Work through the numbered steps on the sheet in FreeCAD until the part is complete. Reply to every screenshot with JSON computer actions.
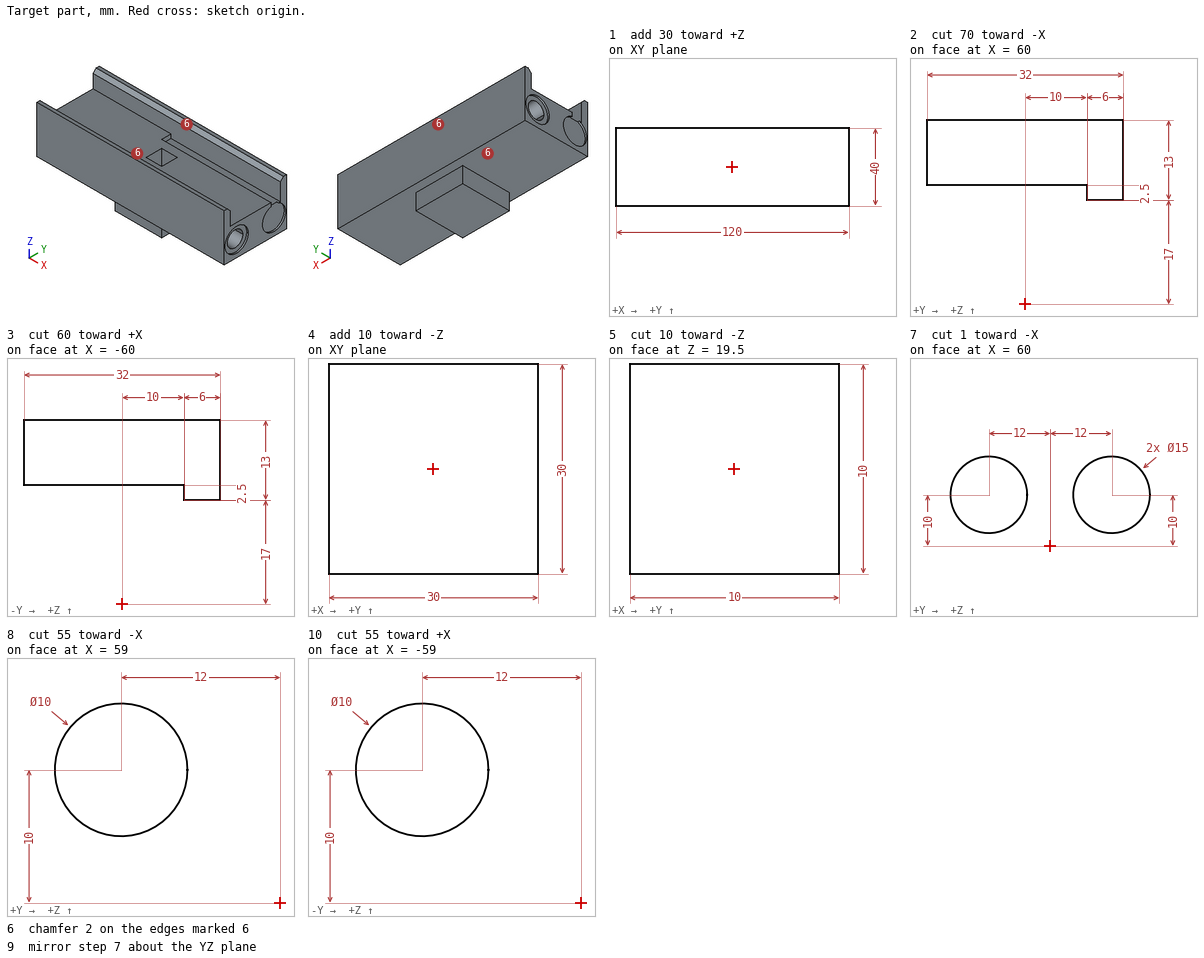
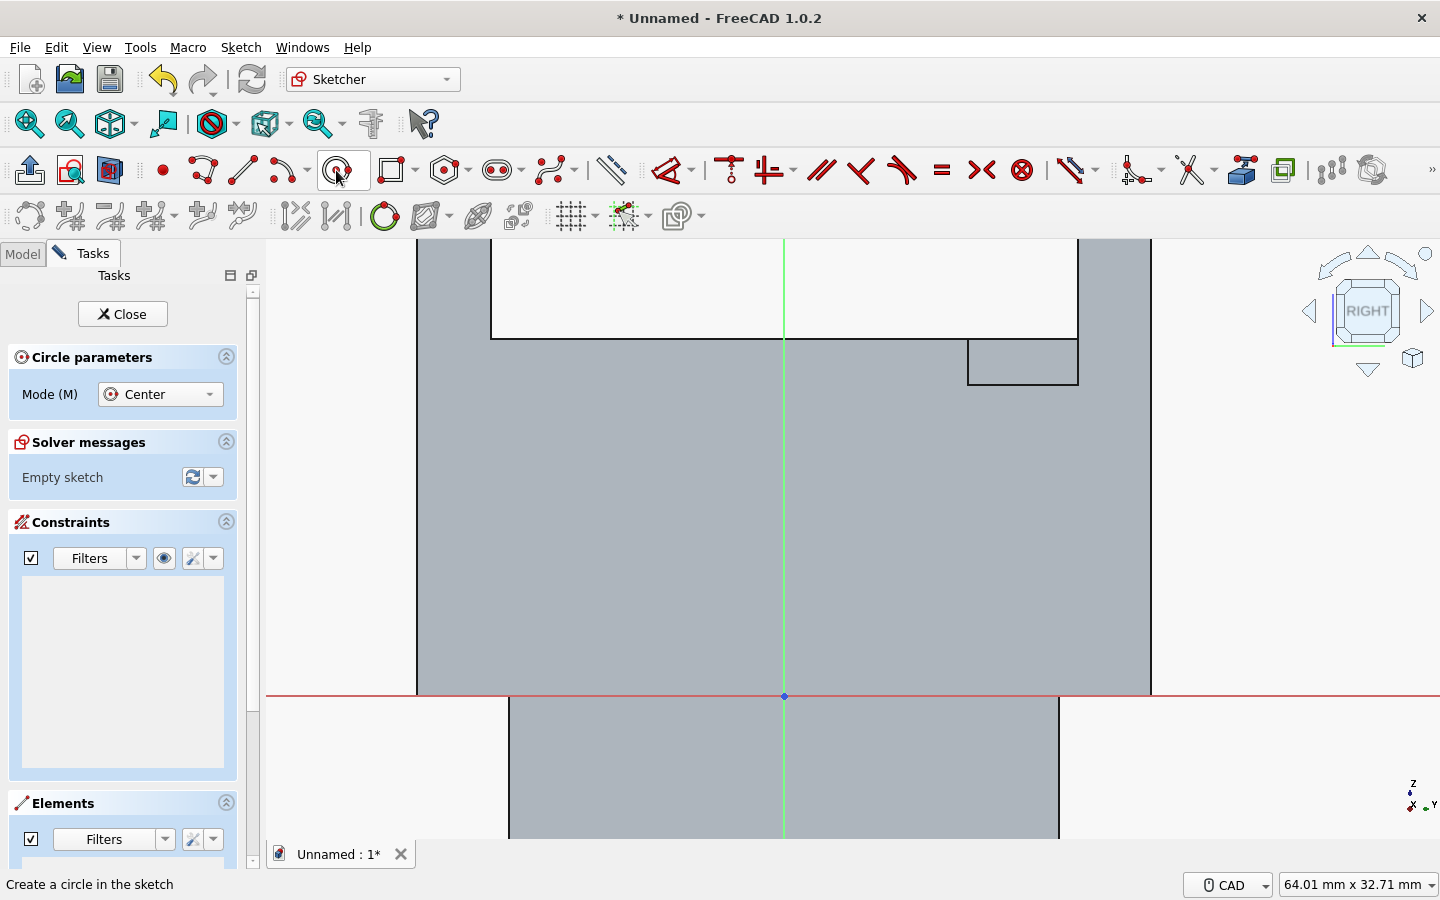
{"action": "left_click", "coordinate": [1004, 513]}
{"action": "mouse_move", "coordinate": [1102, 416]}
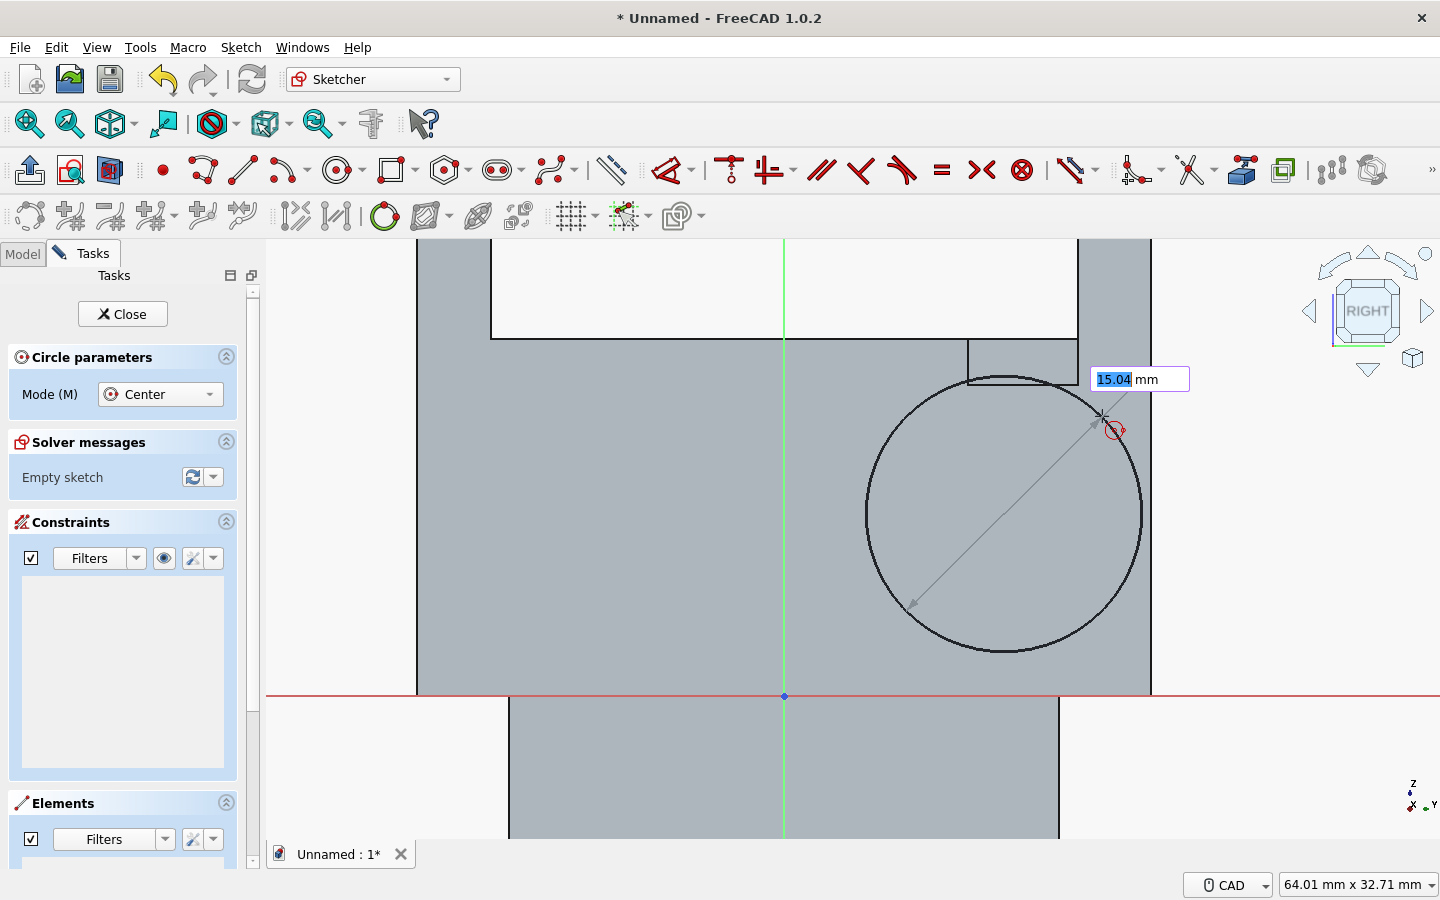
{"action": "type", "text": "15"}
{"action": "key", "text": "Return"}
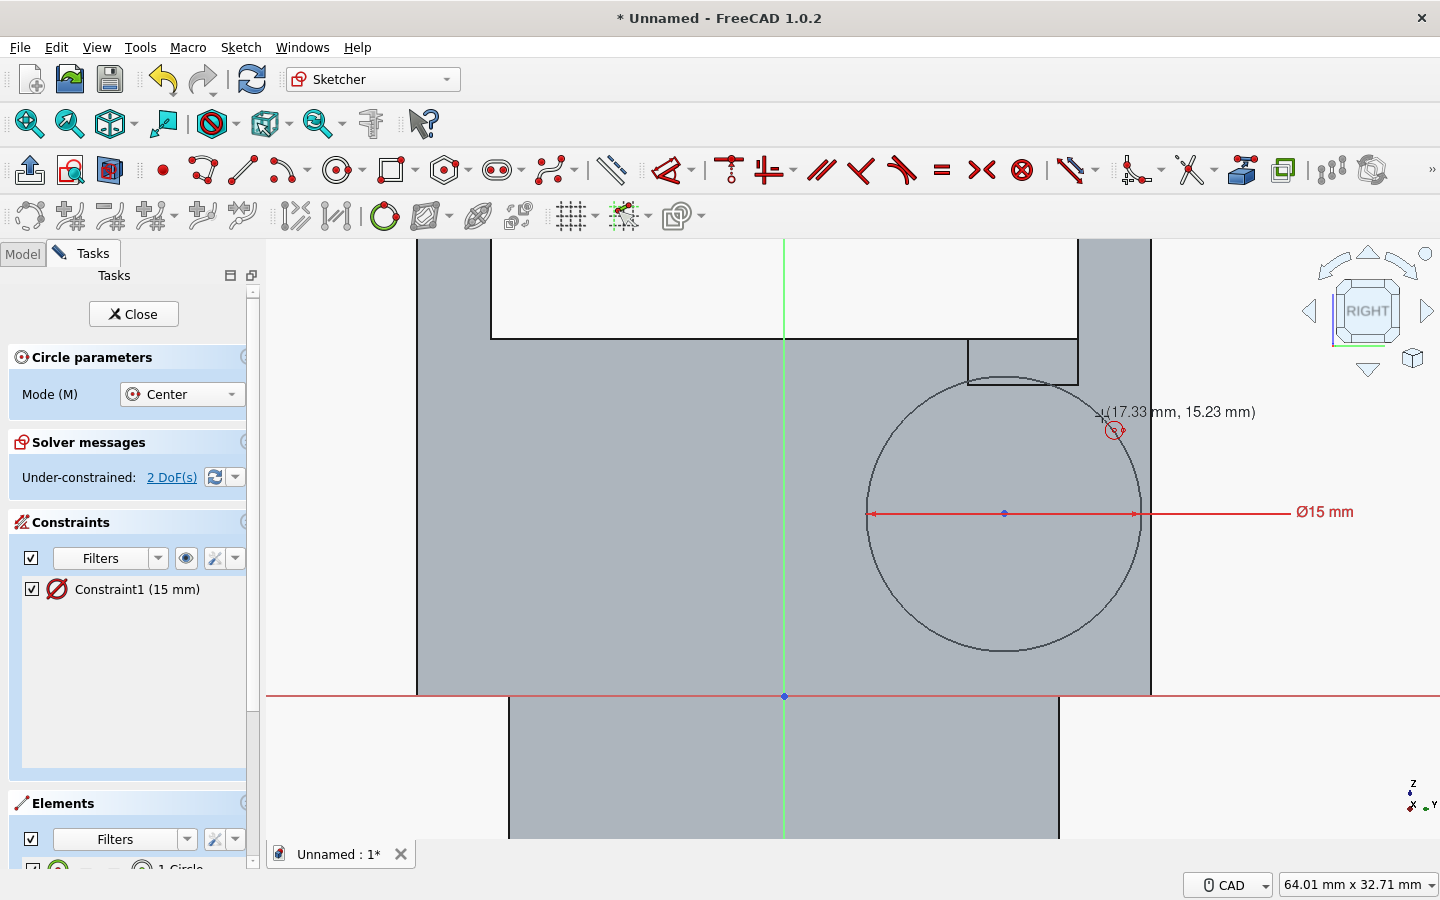
{"action": "left_click", "coordinate": [564, 513]}
{"action": "mouse_move", "coordinate": [661, 416]}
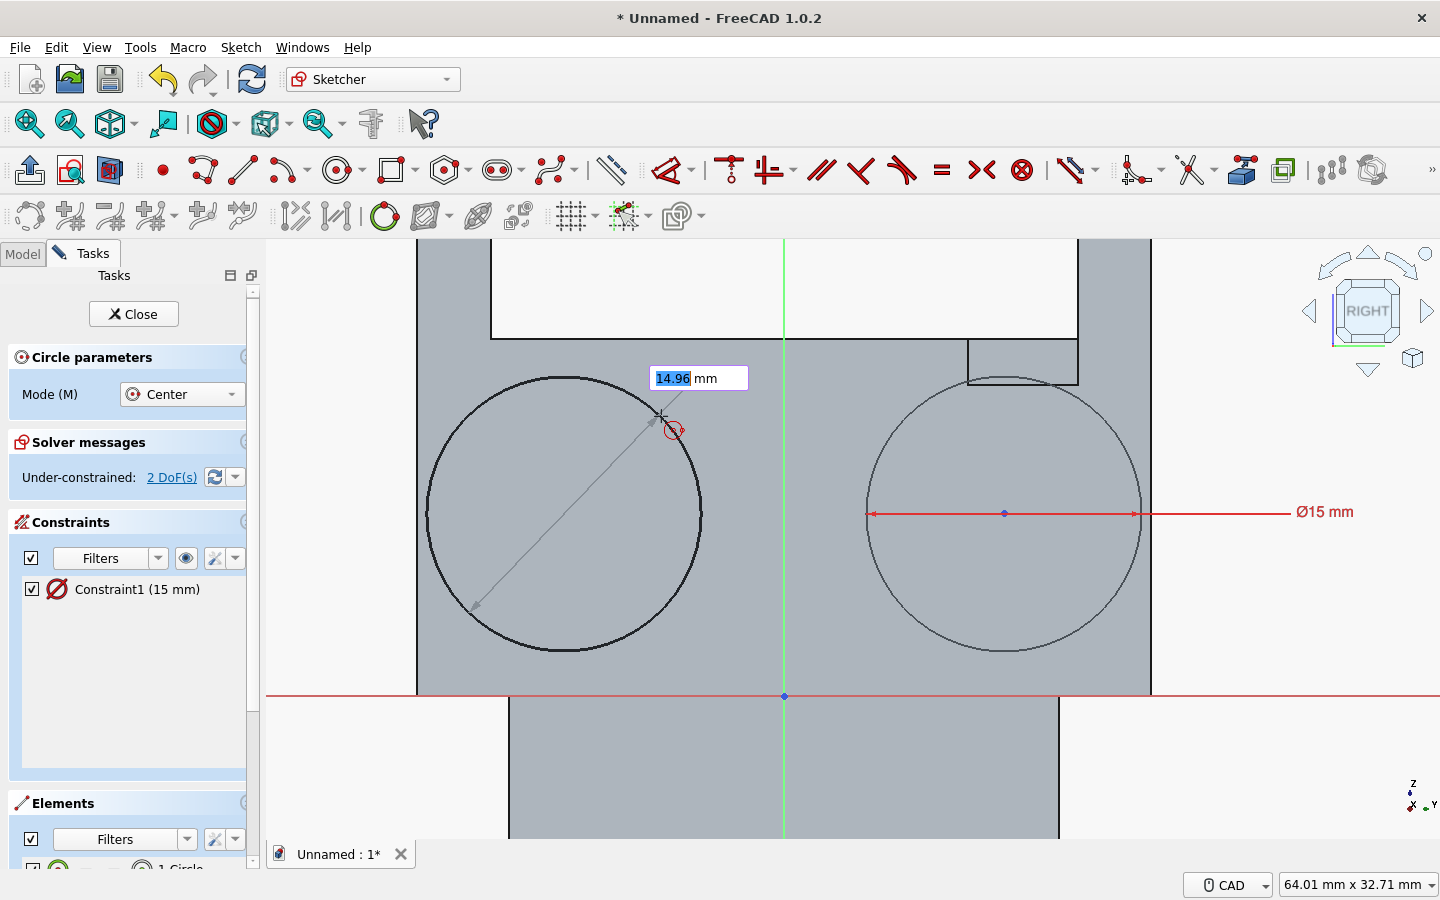
{"action": "type", "text": "15"}
{"action": "key", "text": "Return"}
{"action": "key", "text": "Escape"}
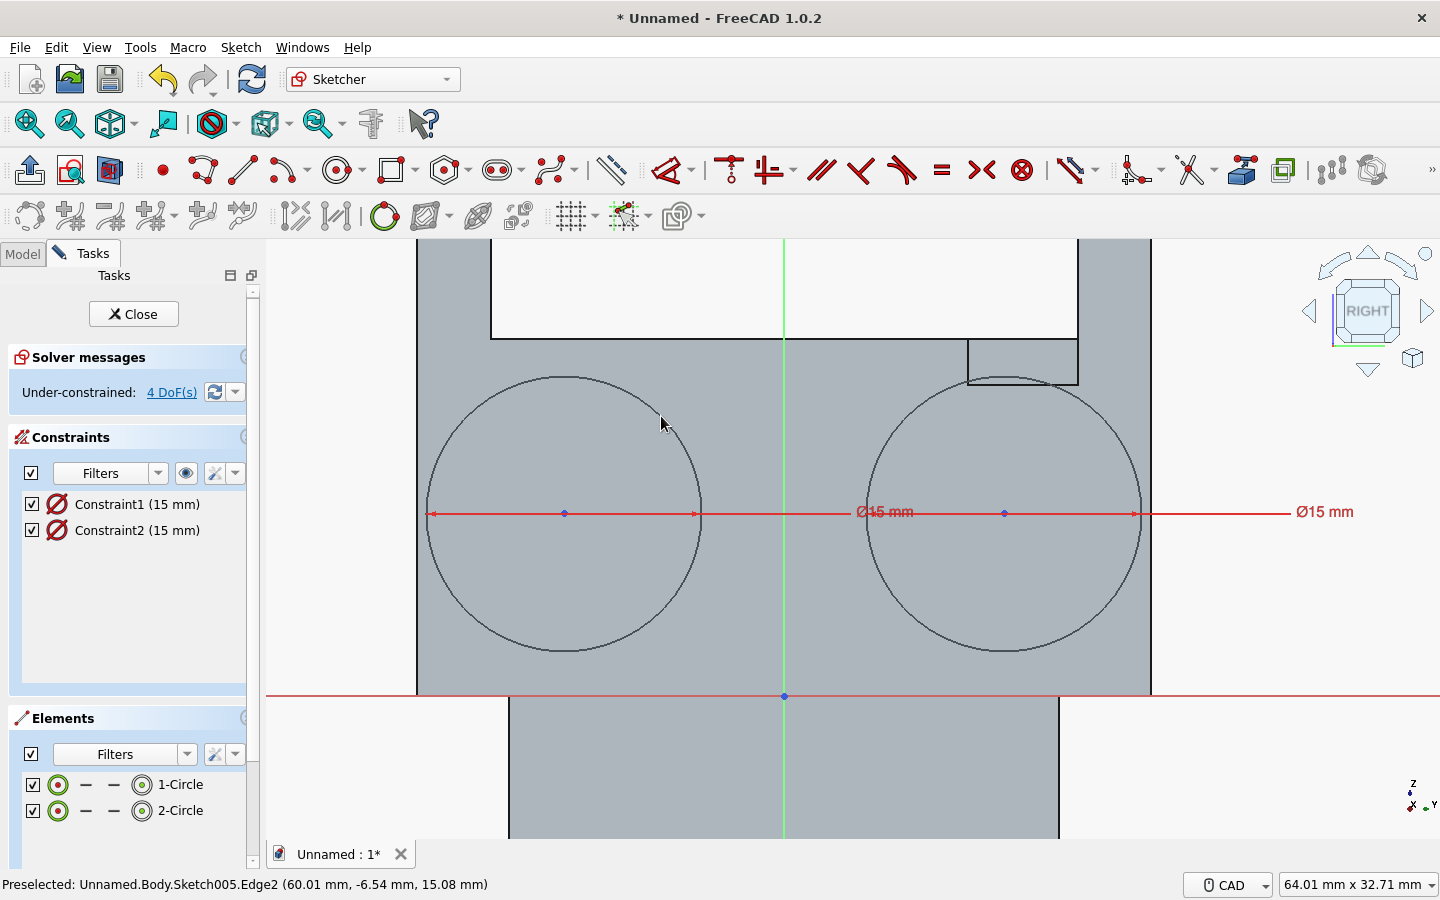
{"action": "key", "text": "d"}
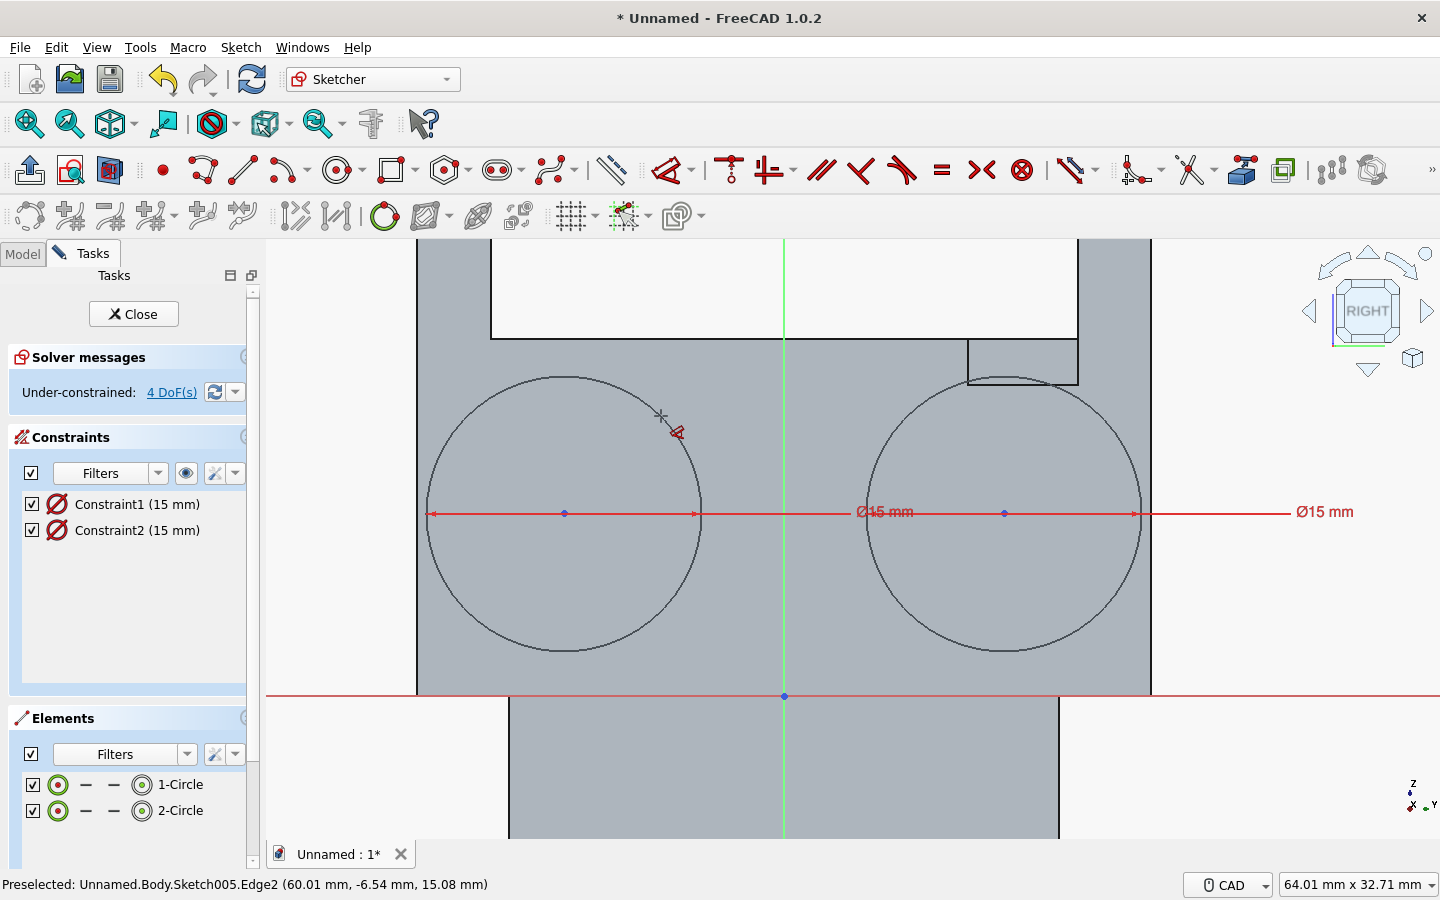
{"action": "left_click", "coordinate": [1004, 514]}
{"action": "left_click", "coordinate": [894, 730]}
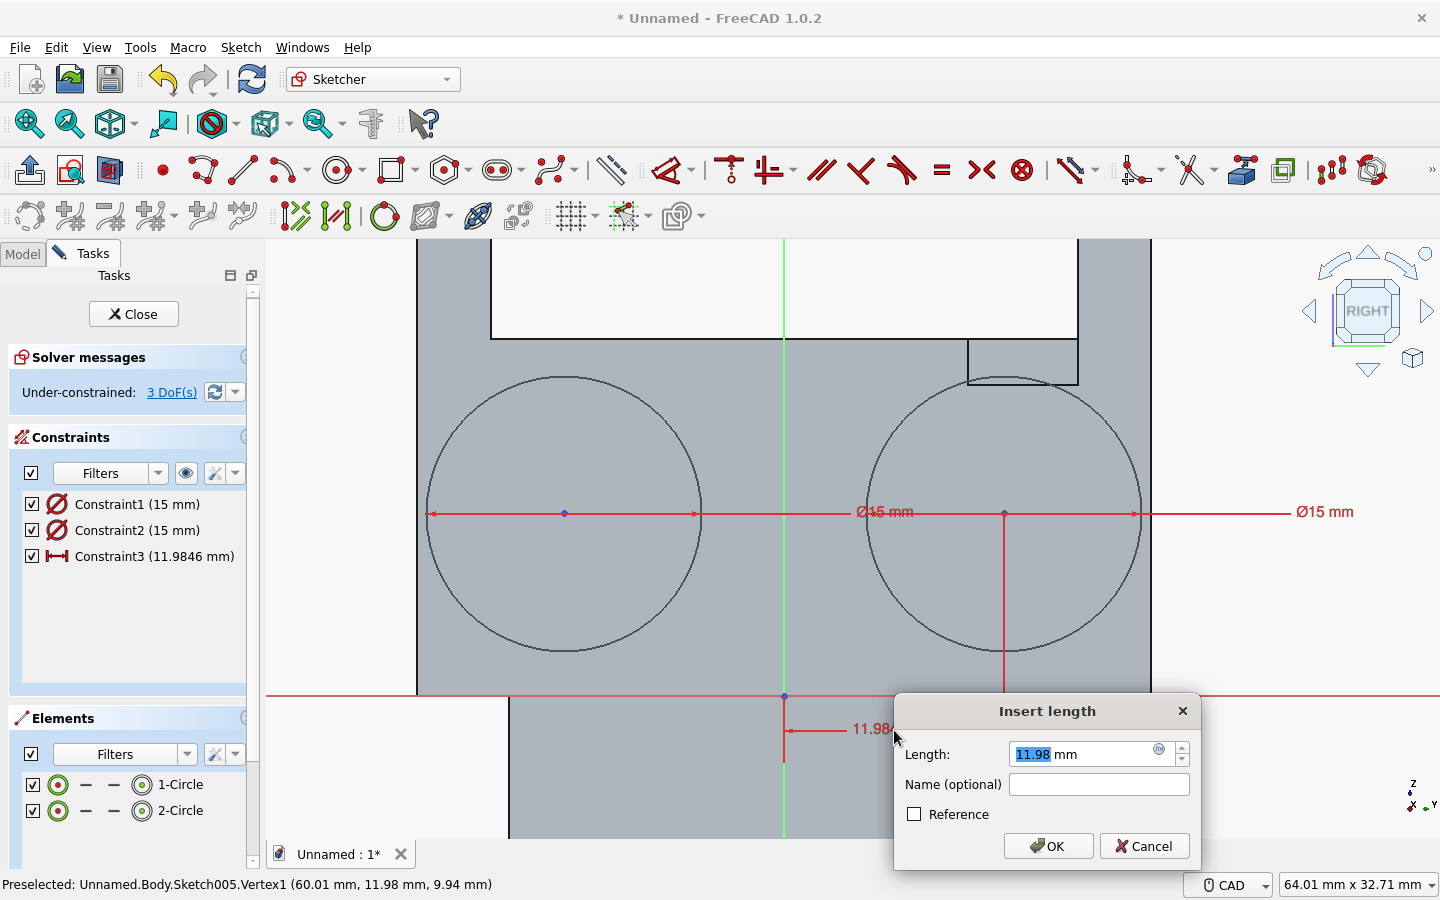
{"action": "type", "text": "12"}
{"action": "key", "text": "Return"}